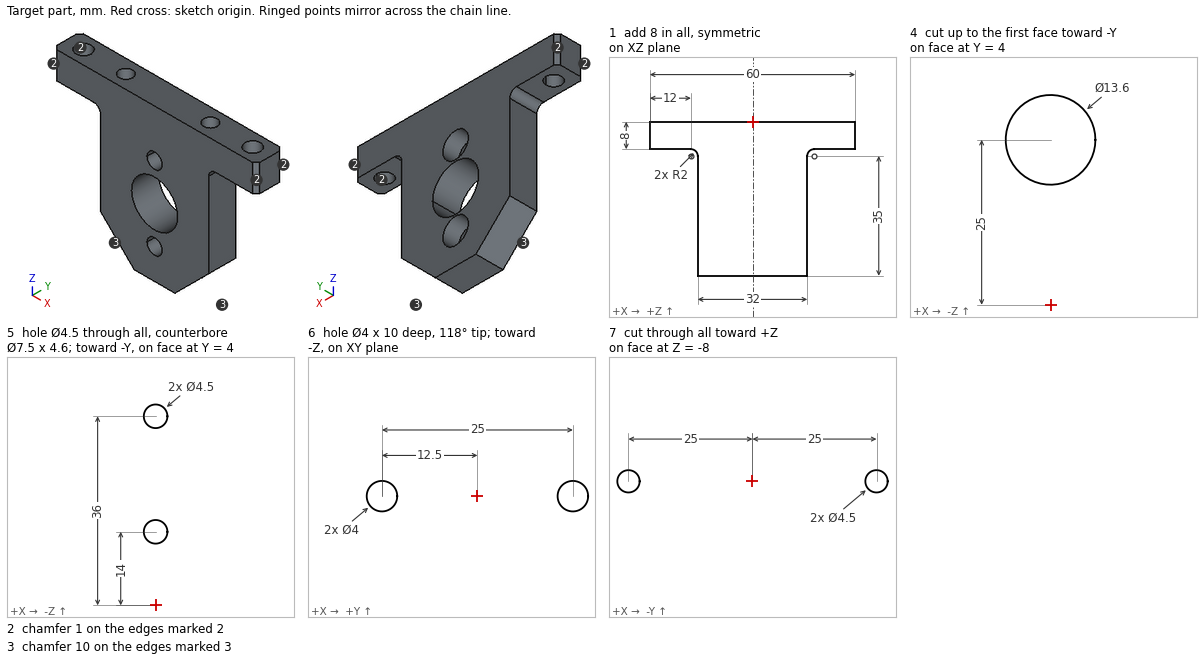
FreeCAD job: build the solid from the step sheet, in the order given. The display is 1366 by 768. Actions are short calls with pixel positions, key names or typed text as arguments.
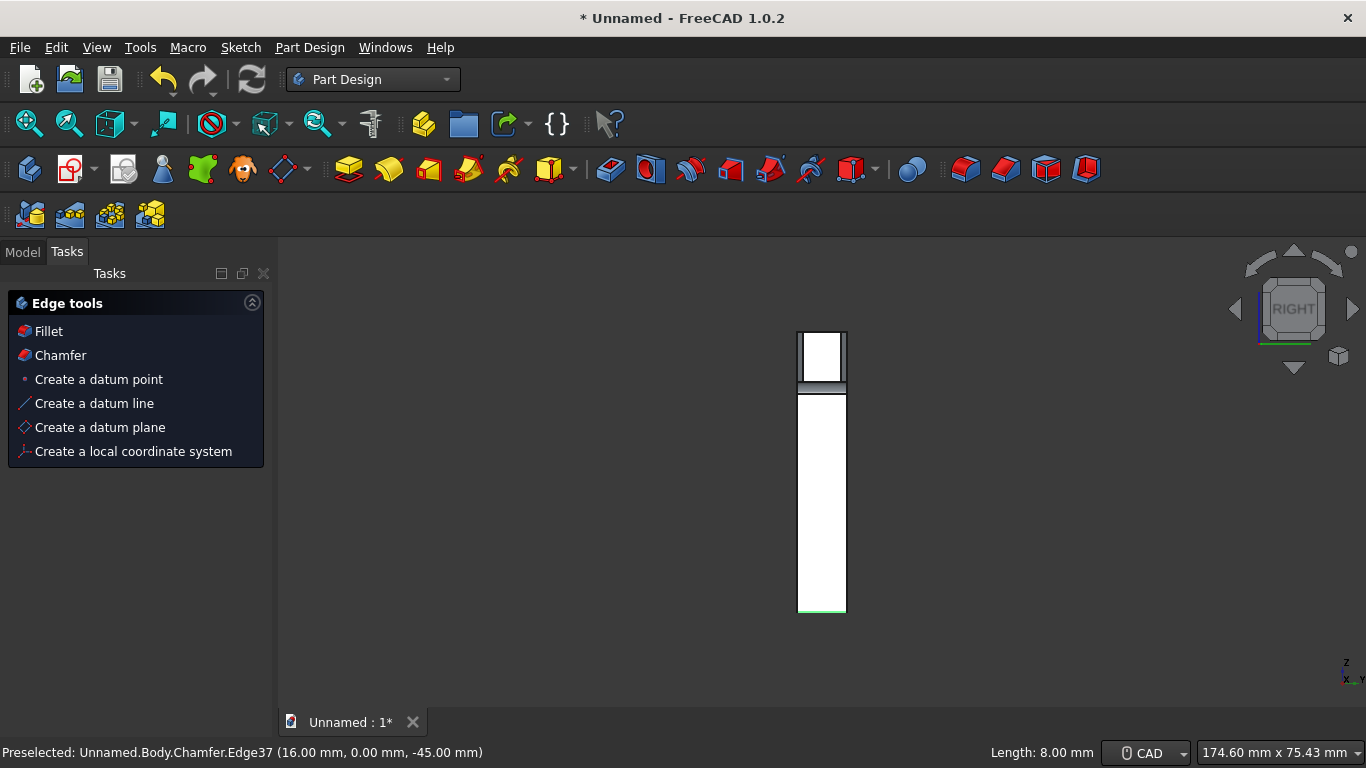
key(5)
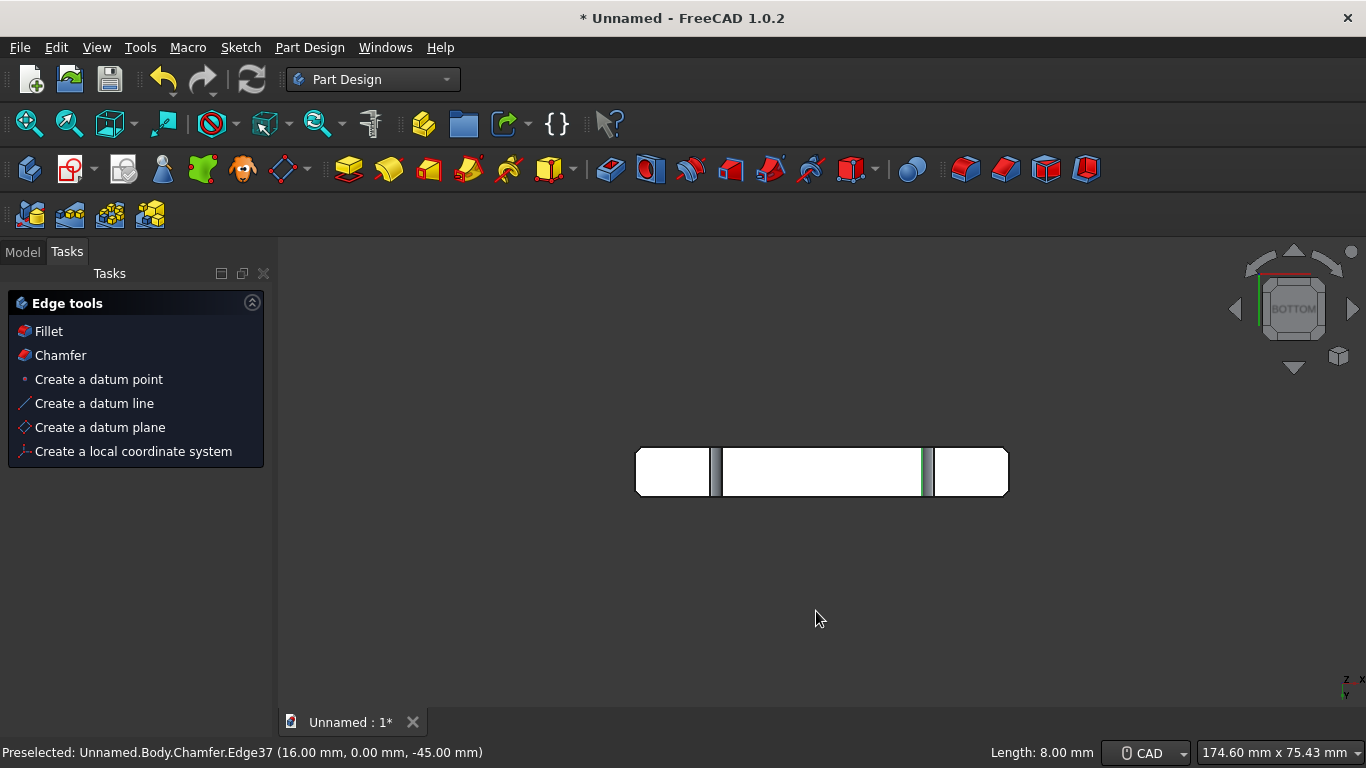
click(30, 124)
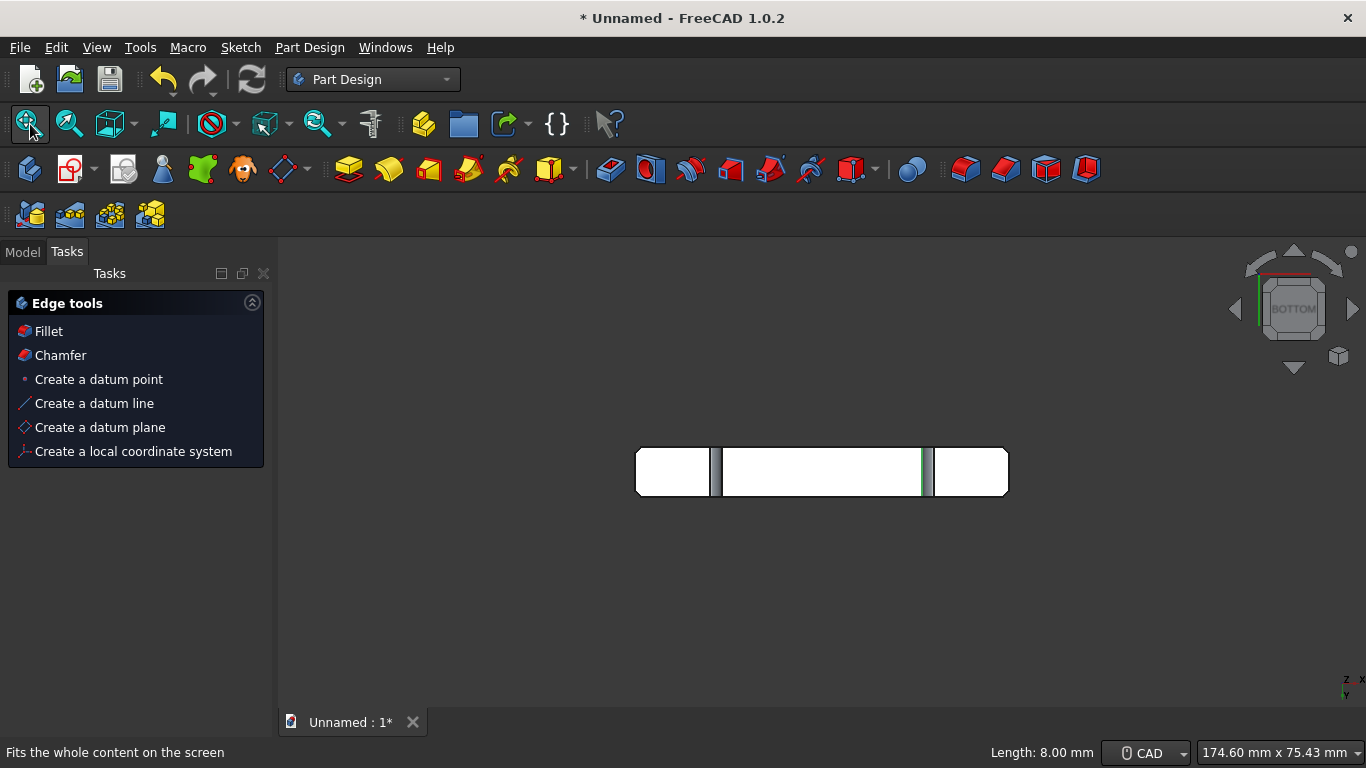
click(722, 471, ctrl)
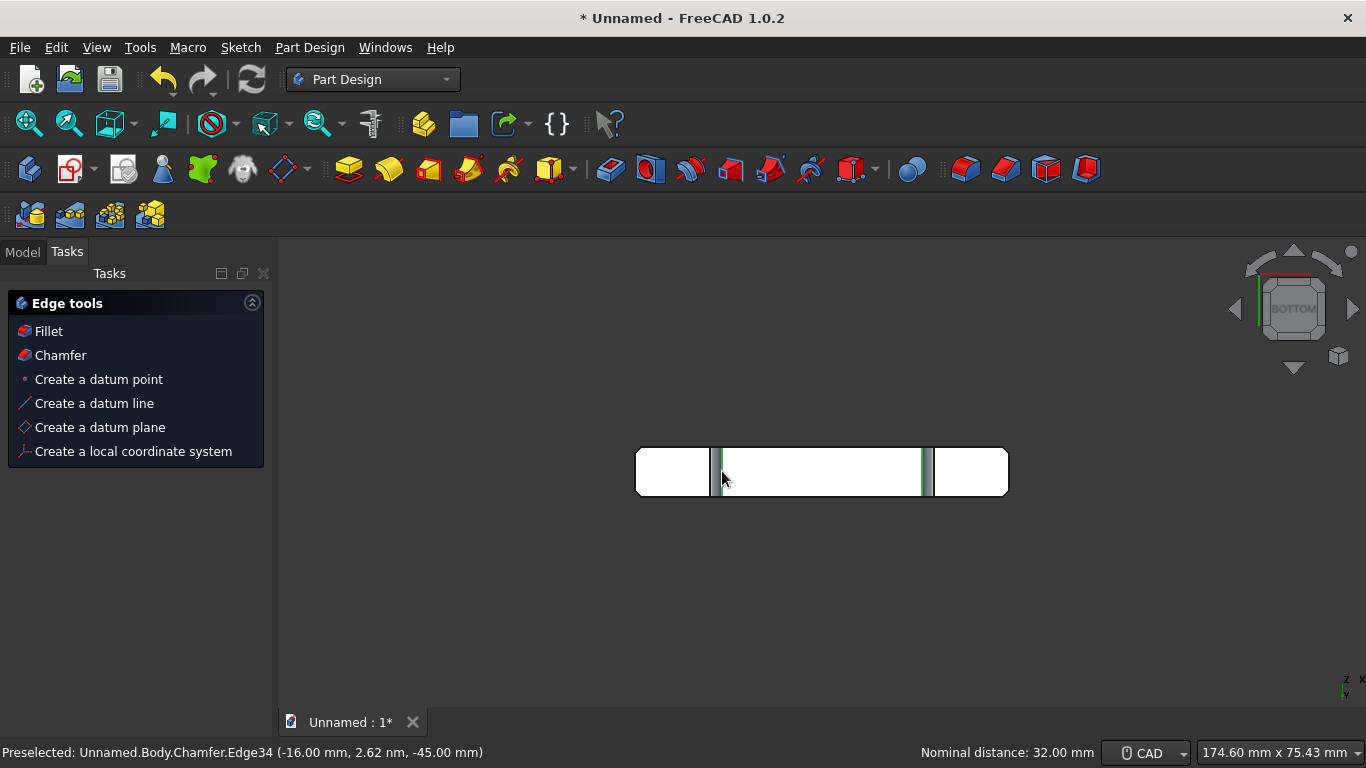
click(1006, 170)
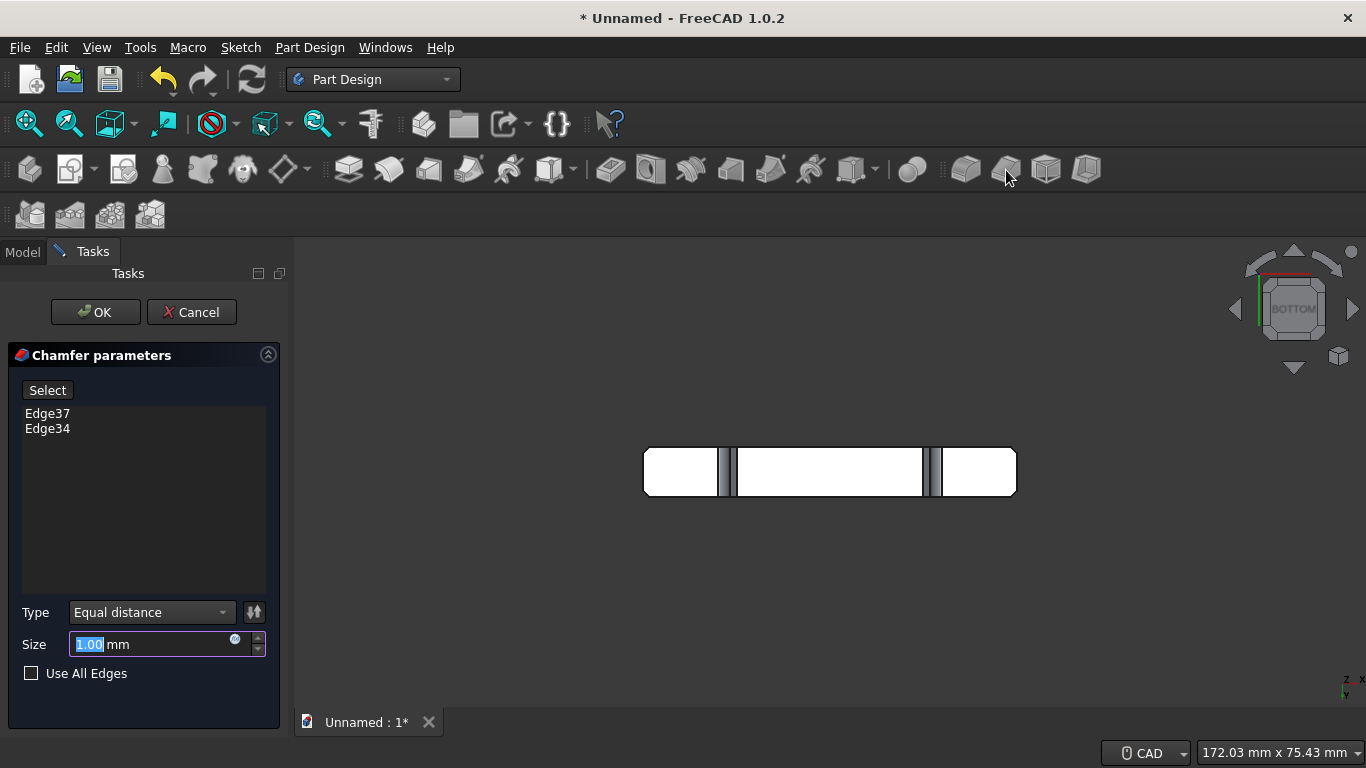
text(10)
key(Tab)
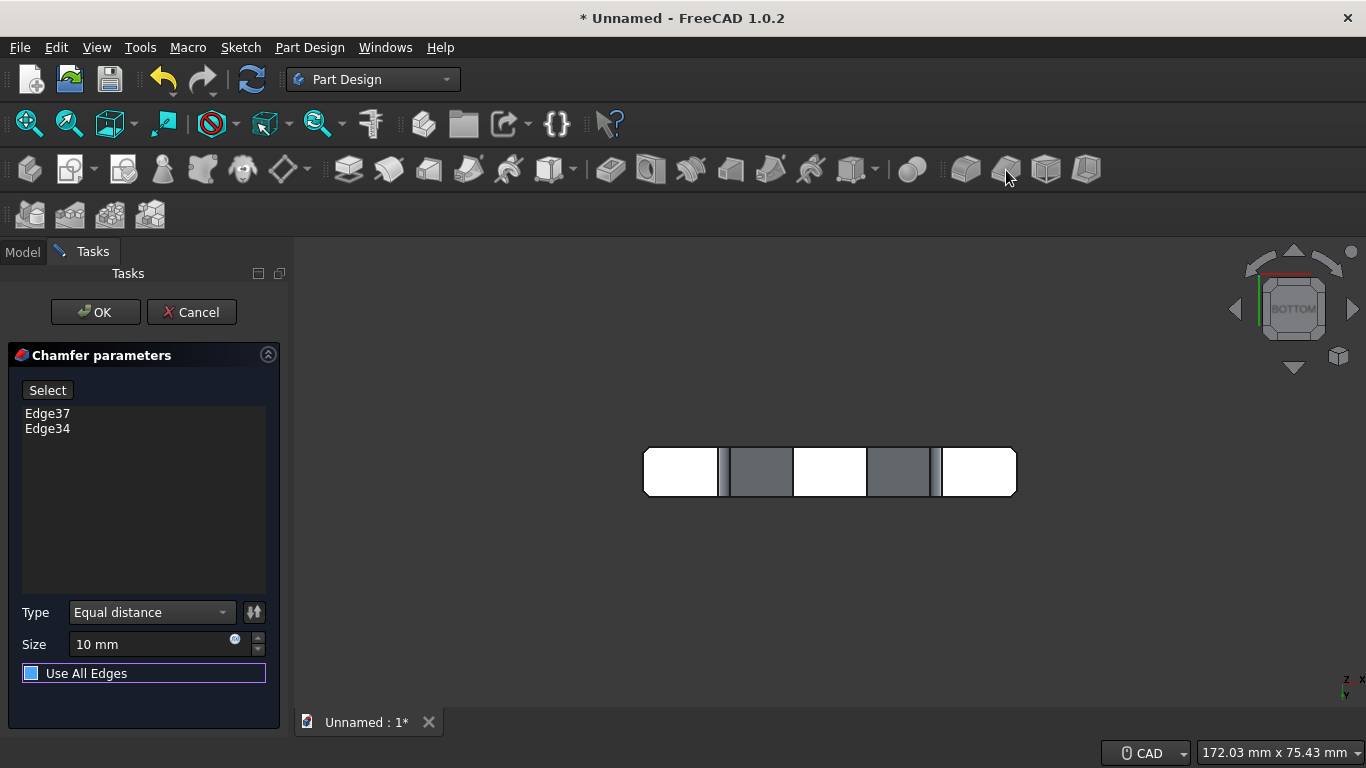
click(96, 312)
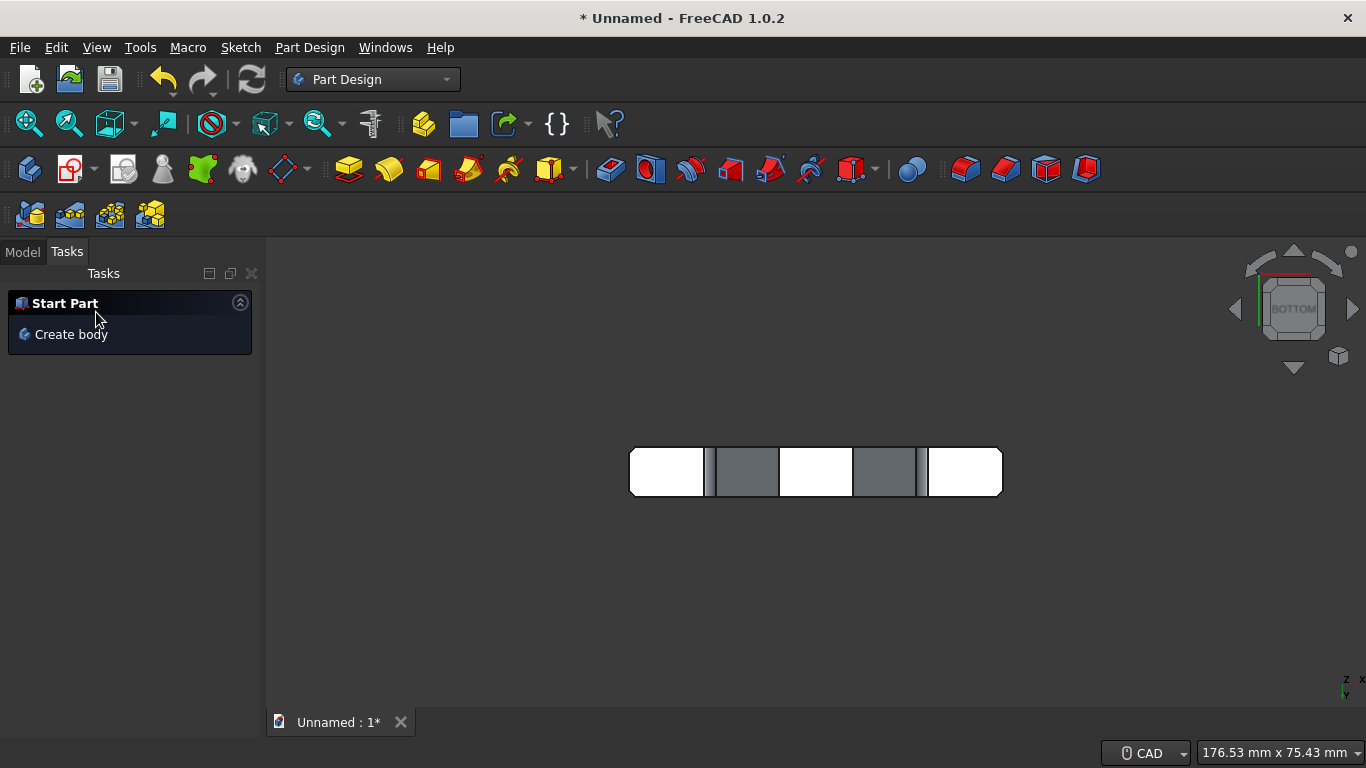
click(30, 124)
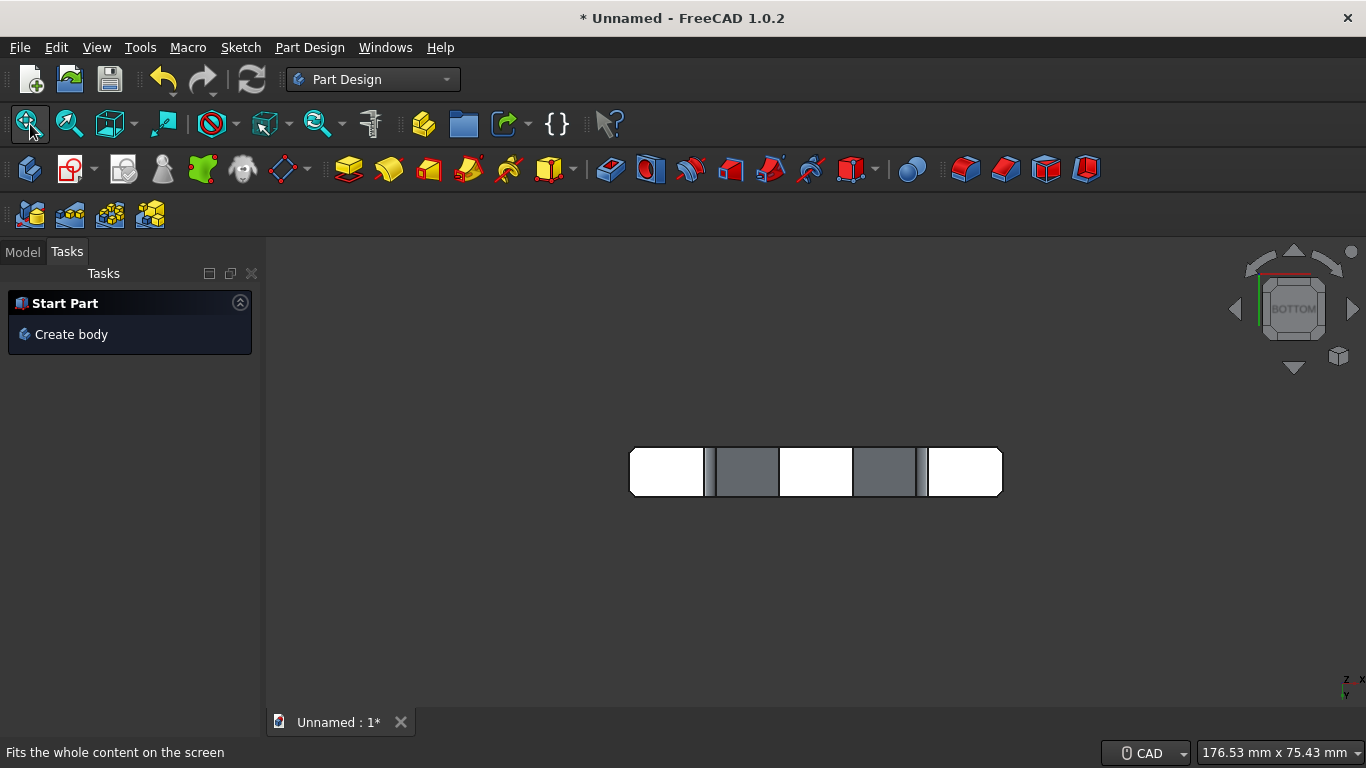
key(4)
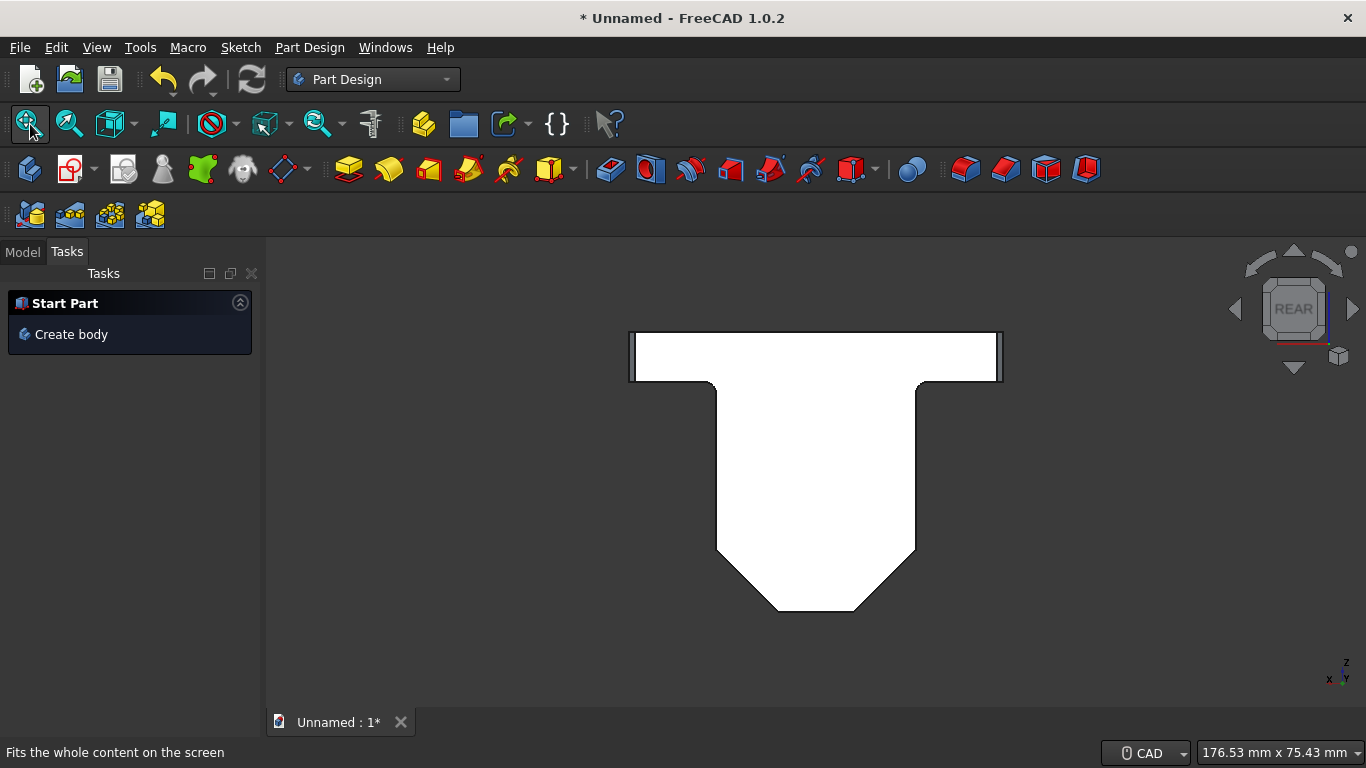
click(816, 431)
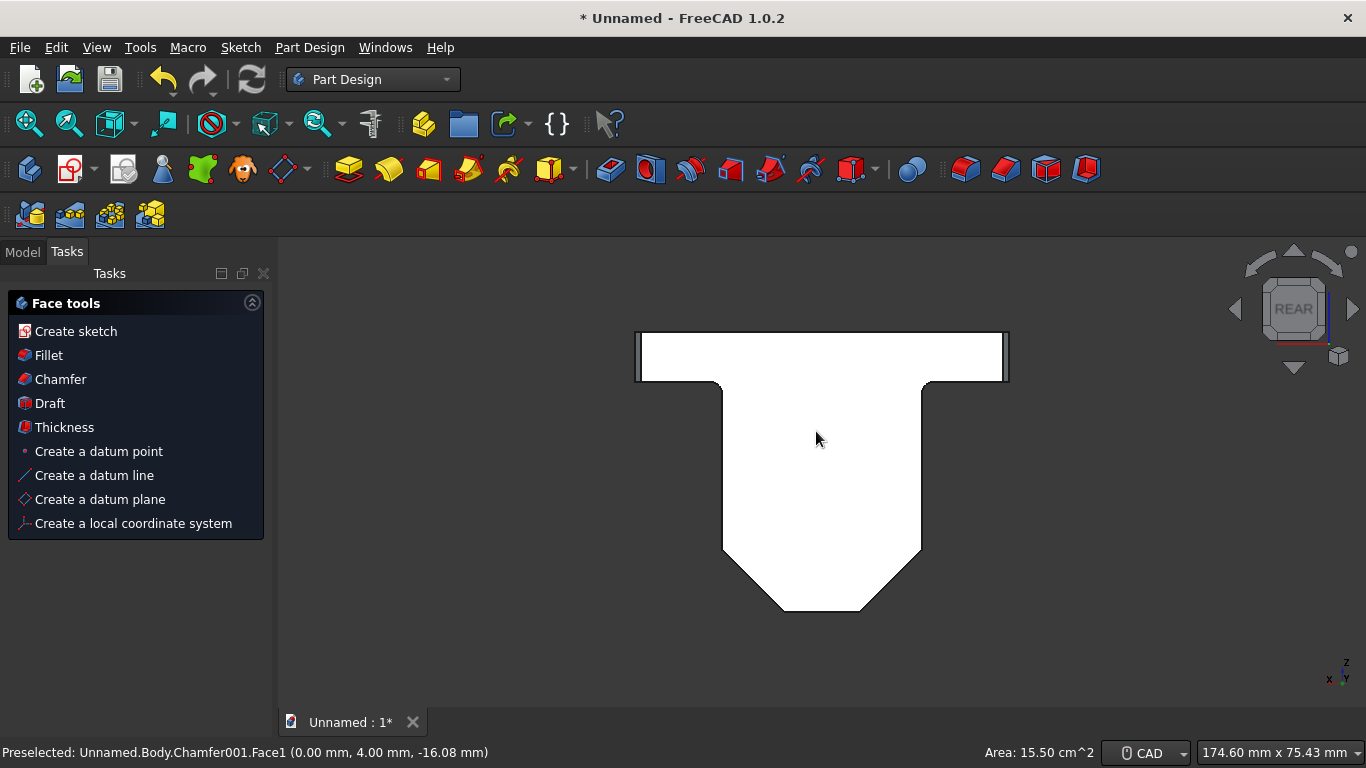
click(70, 170)